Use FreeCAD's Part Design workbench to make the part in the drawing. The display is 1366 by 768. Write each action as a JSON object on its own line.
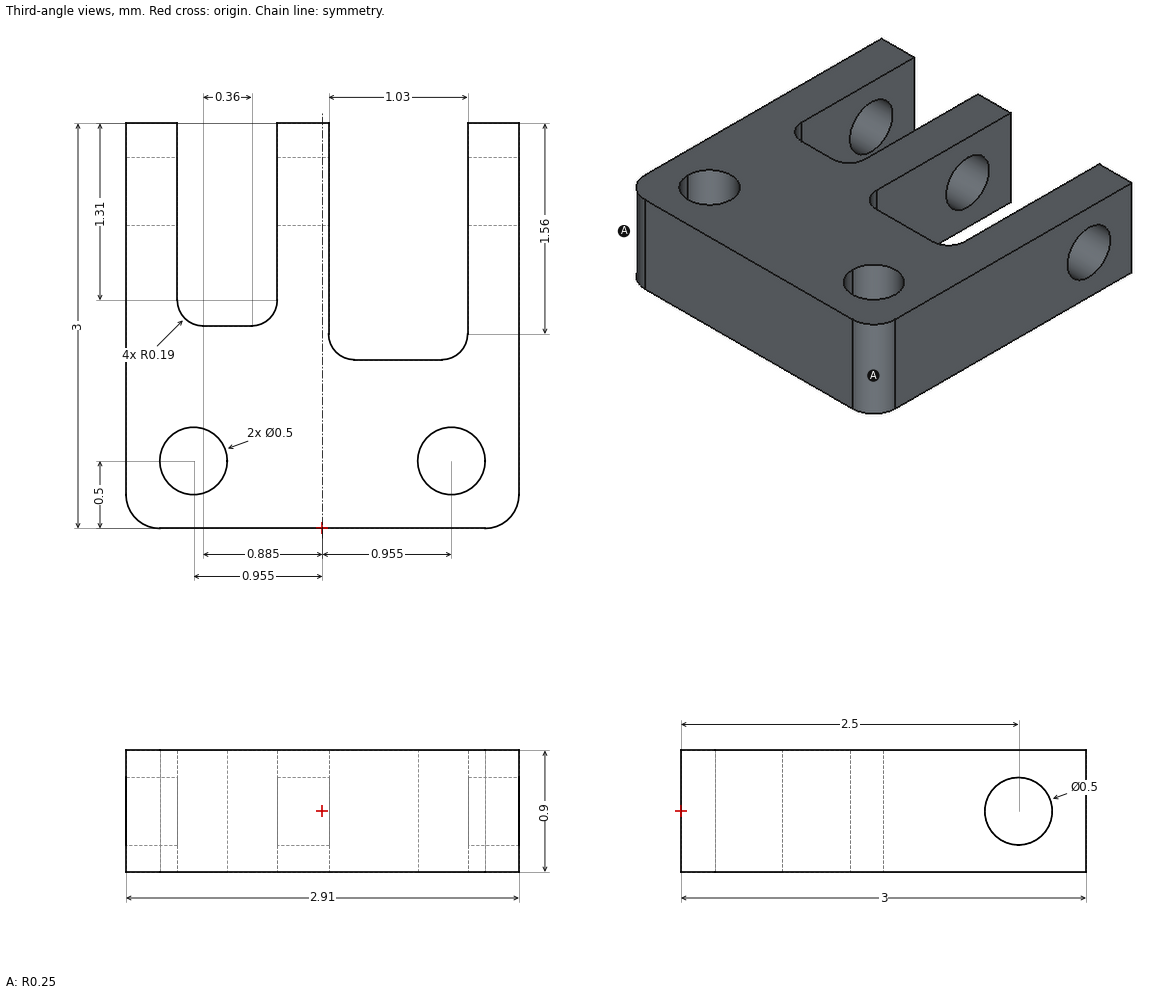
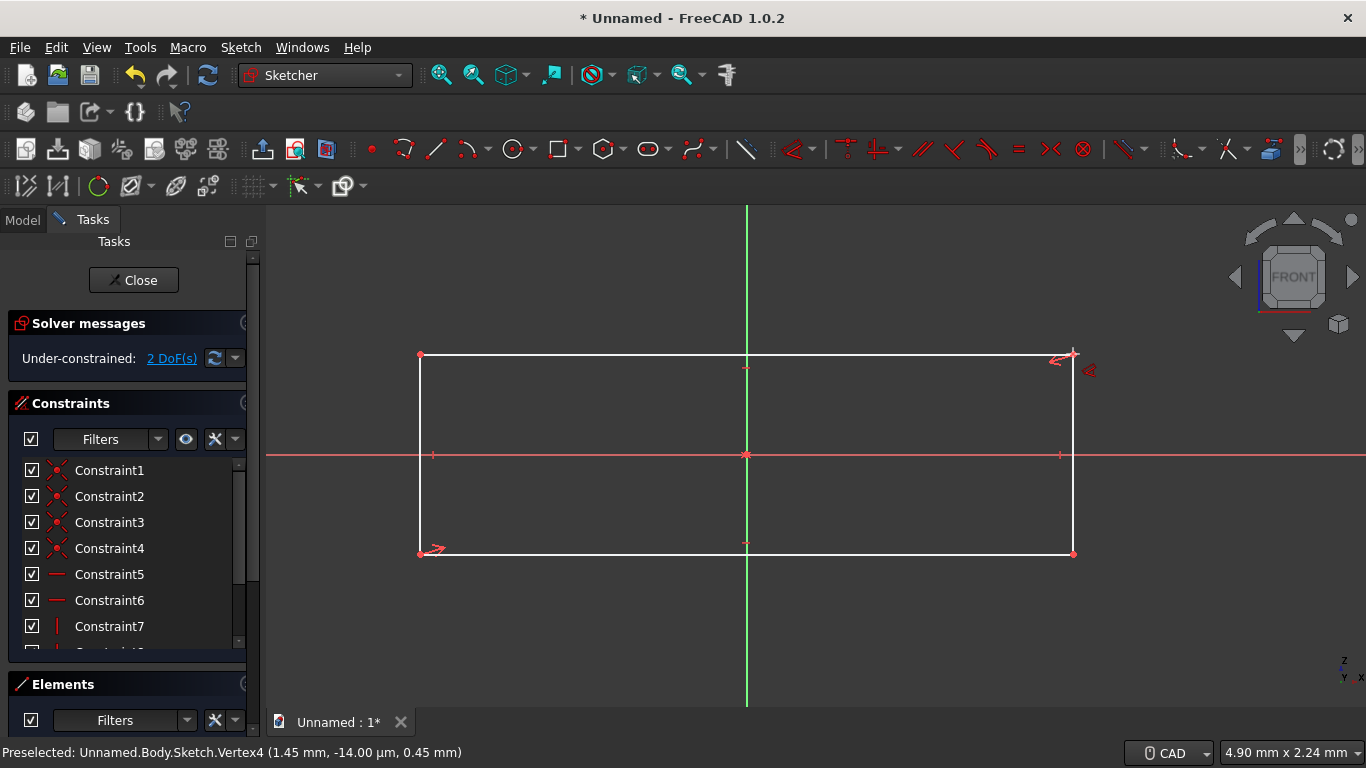
{"action": "left_click", "coordinate": [1073, 495]}
{"action": "left_click", "coordinate": [1107, 409]}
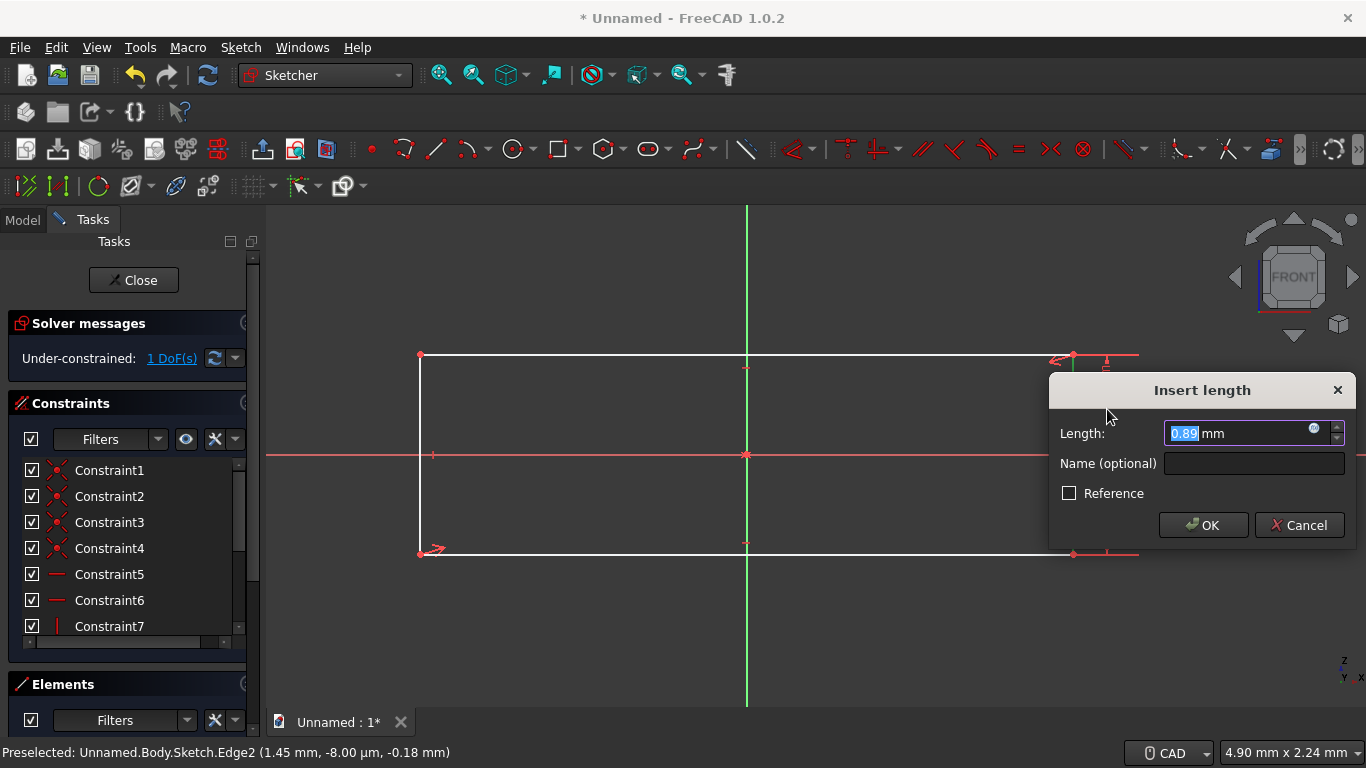
{"action": "type", "text": "0.9"}
{"action": "key", "text": "Return"}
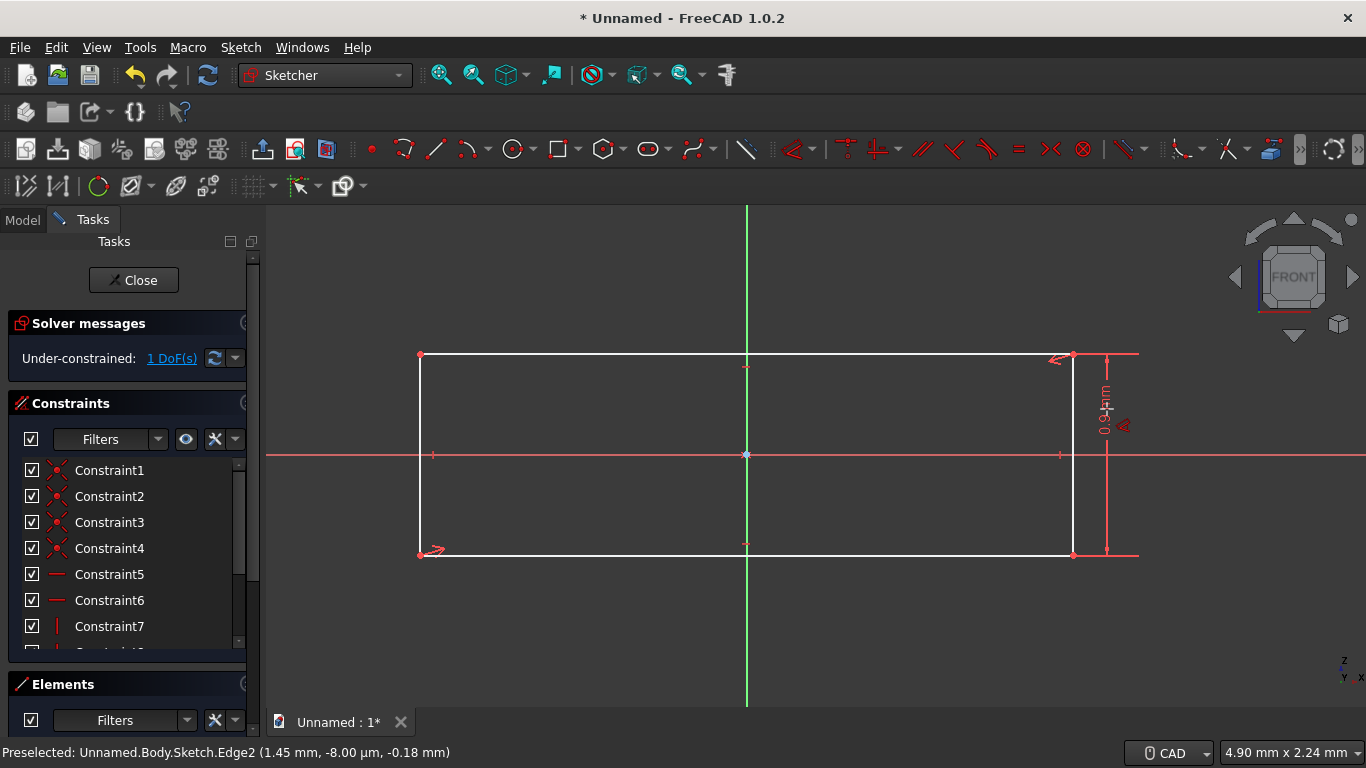
{"action": "left_click", "coordinate": [616, 556]}
{"action": "left_click", "coordinate": [597, 590]}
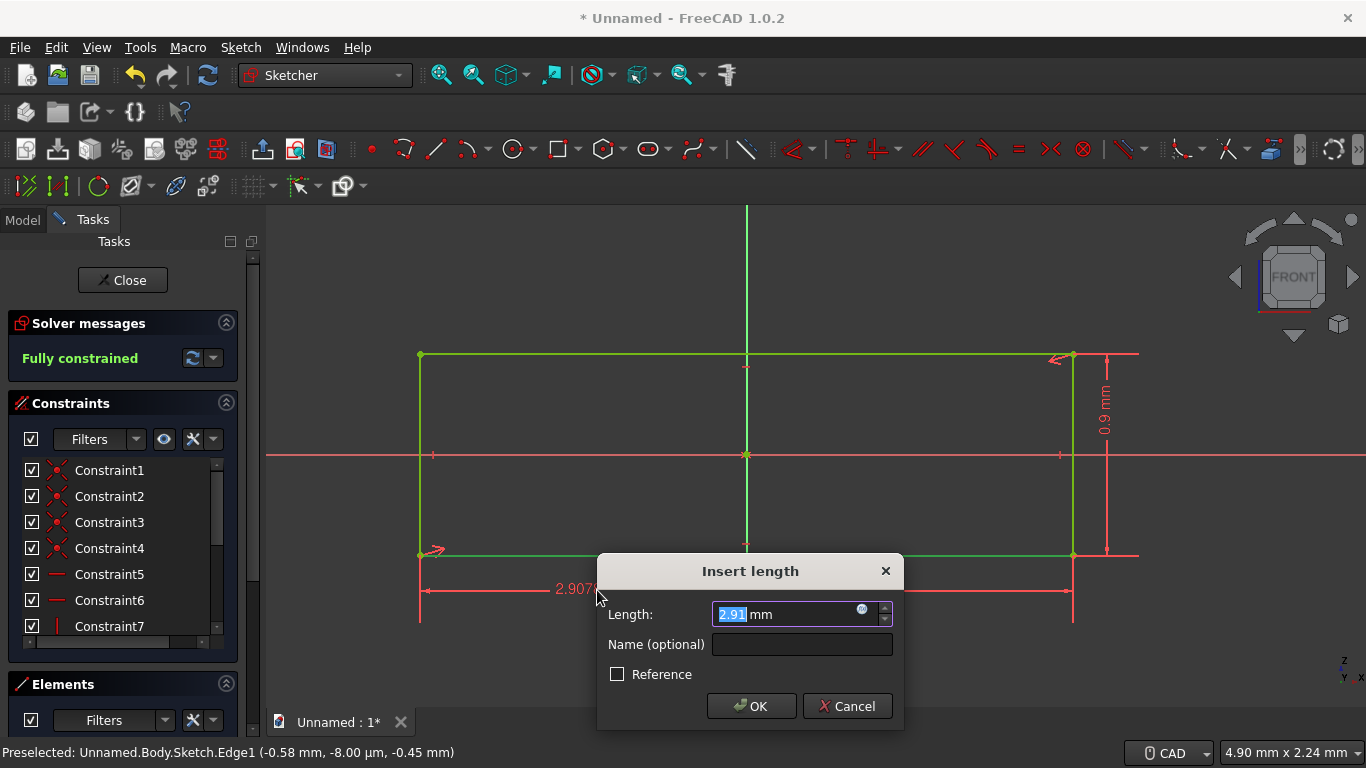
{"action": "type", "text": "2.91"}
{"action": "key", "text": "Return"}
{"action": "key", "text": "Escape"}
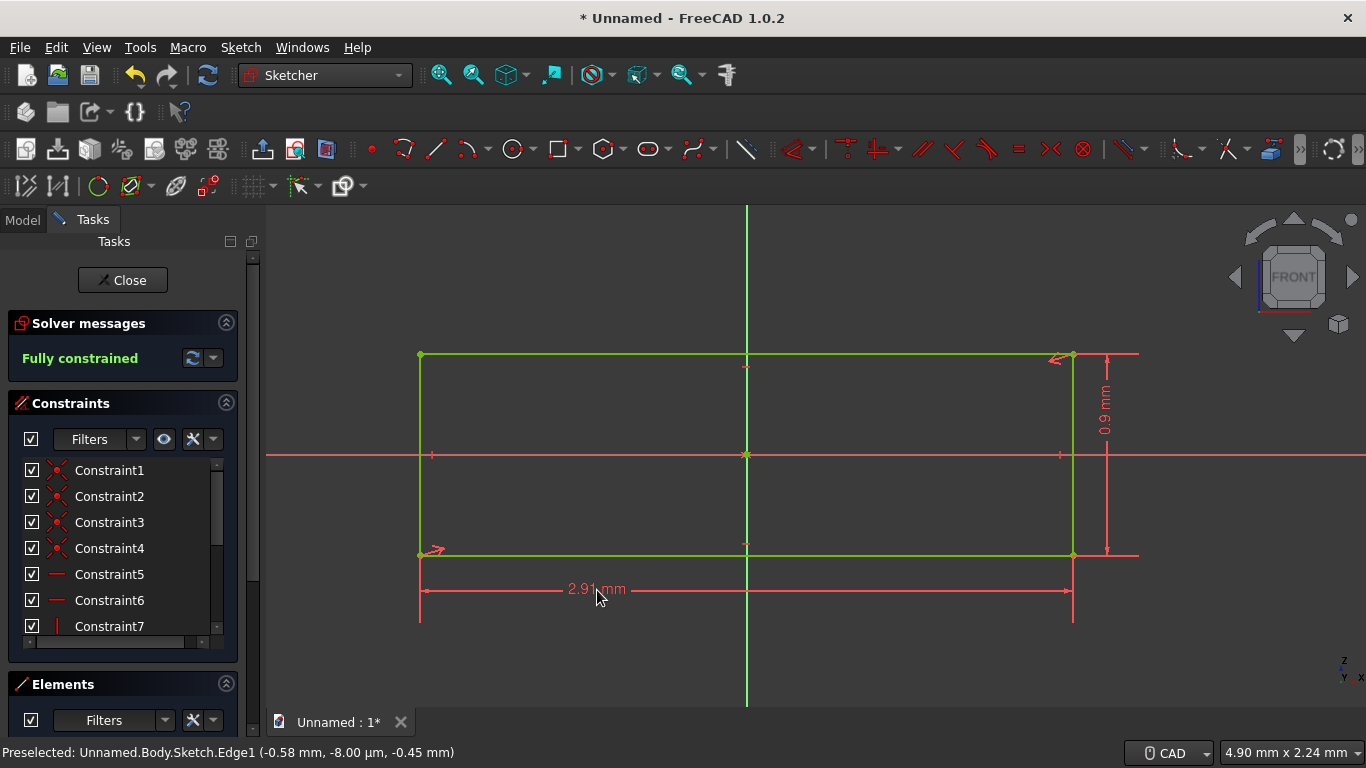
{"action": "left_click", "coordinate": [123, 280]}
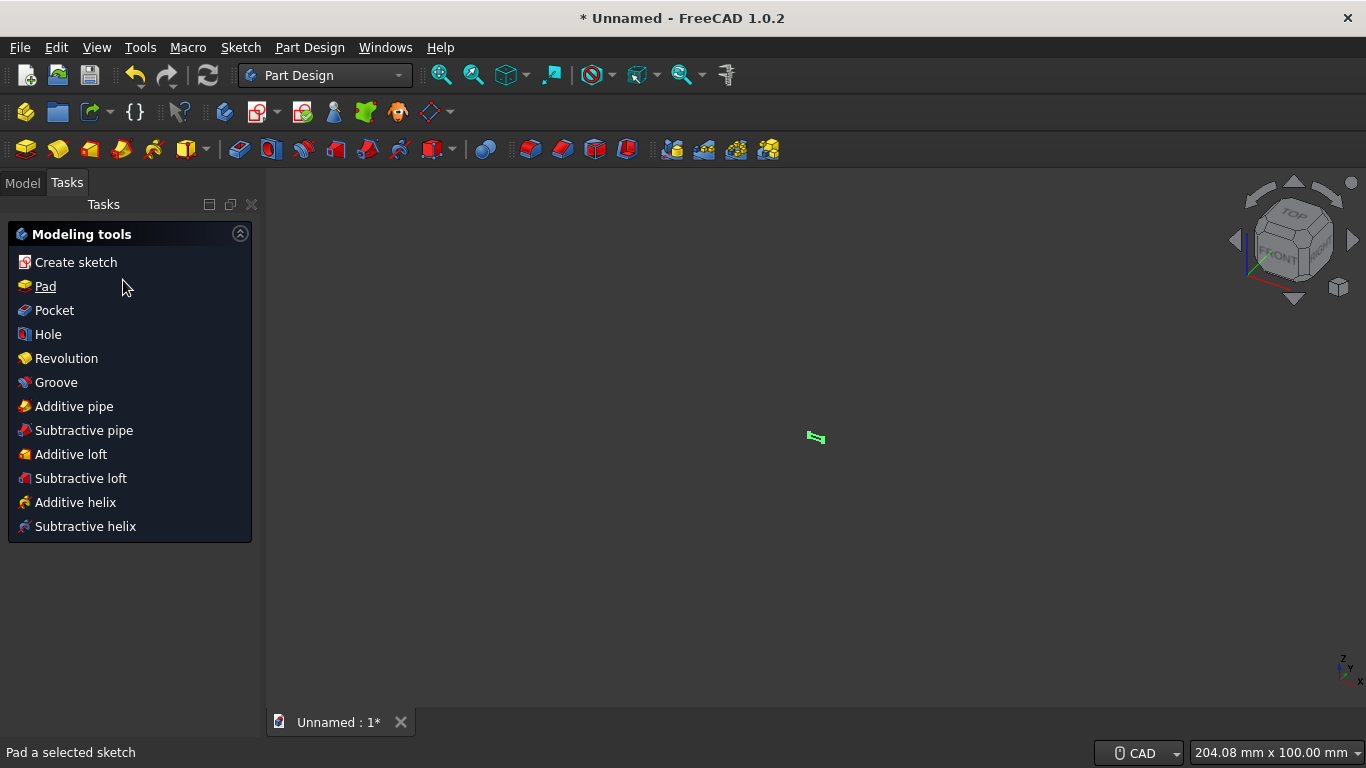
{"action": "left_click", "coordinate": [26, 150]}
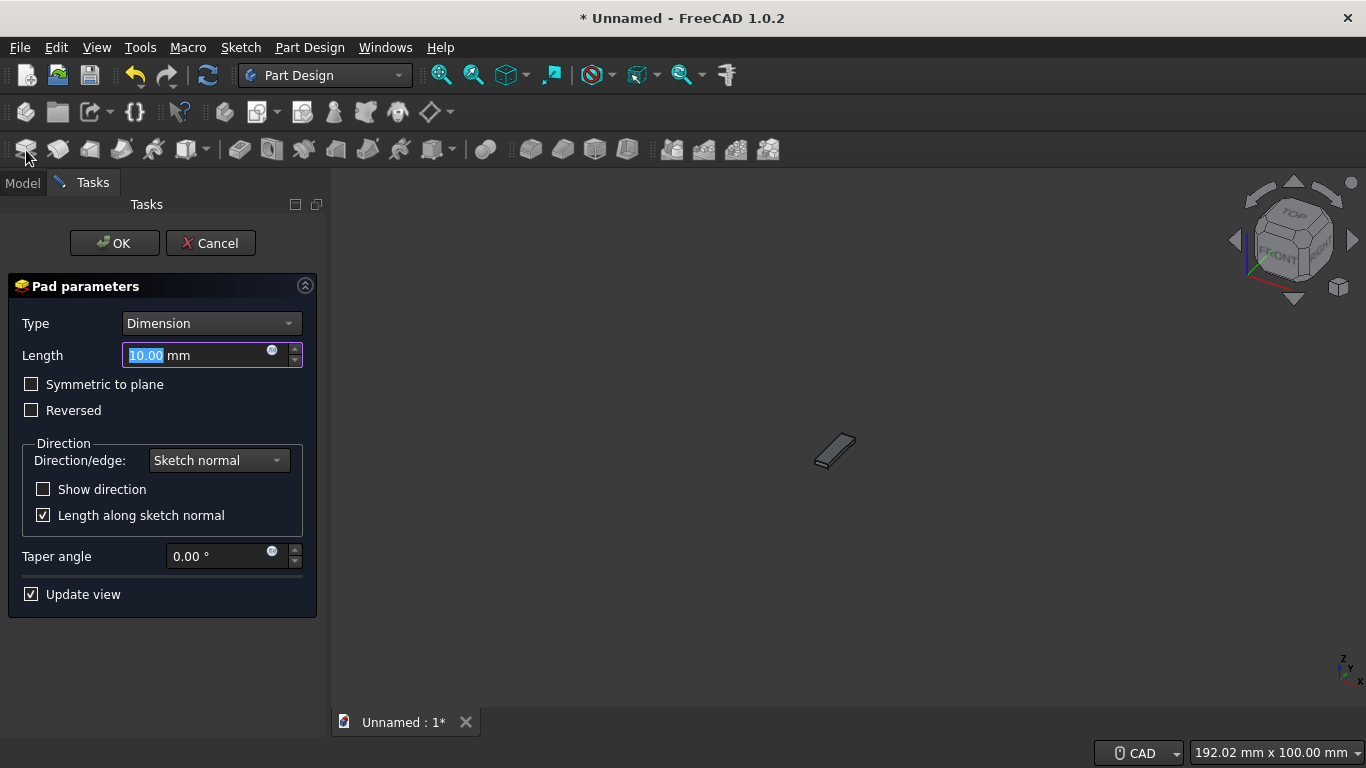
{"action": "type", "text": "3"}
{"action": "key", "text": "Tab"}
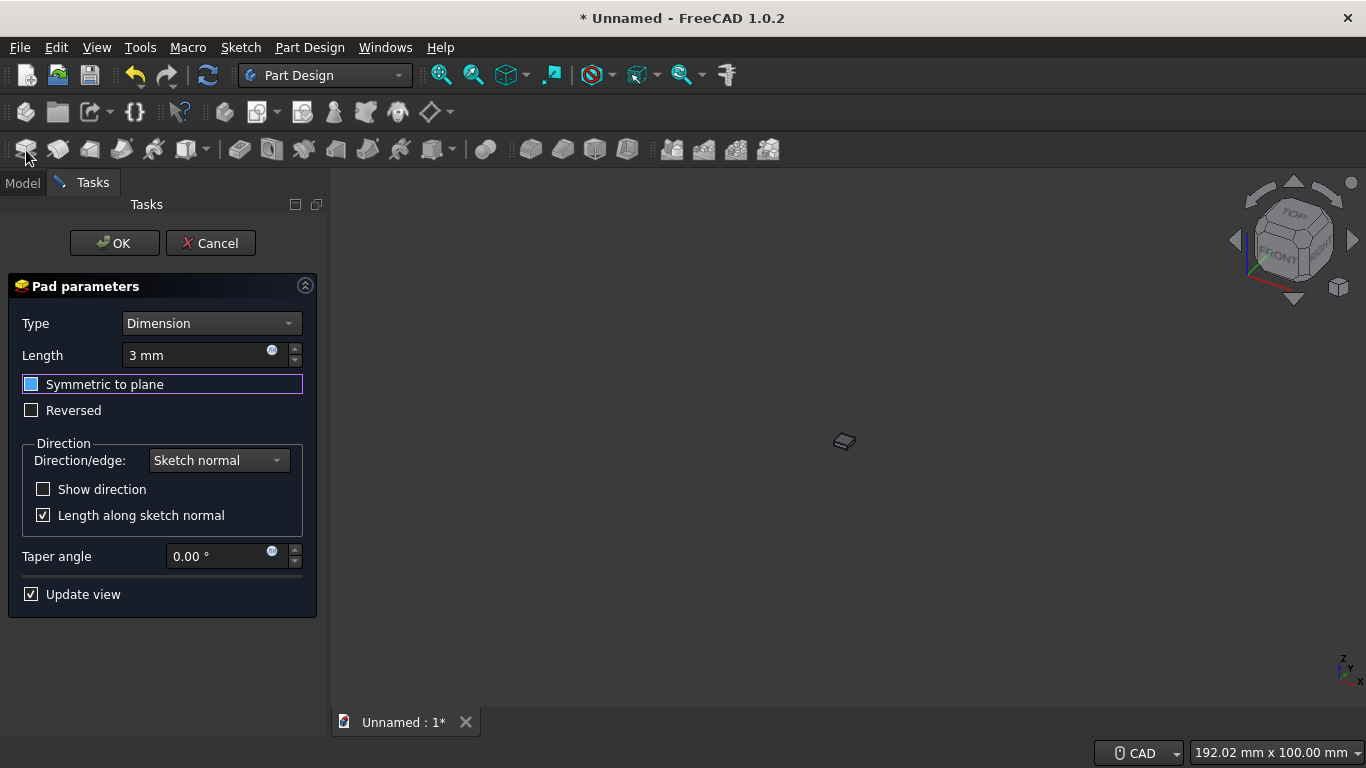
{"action": "left_click", "coordinate": [30, 410]}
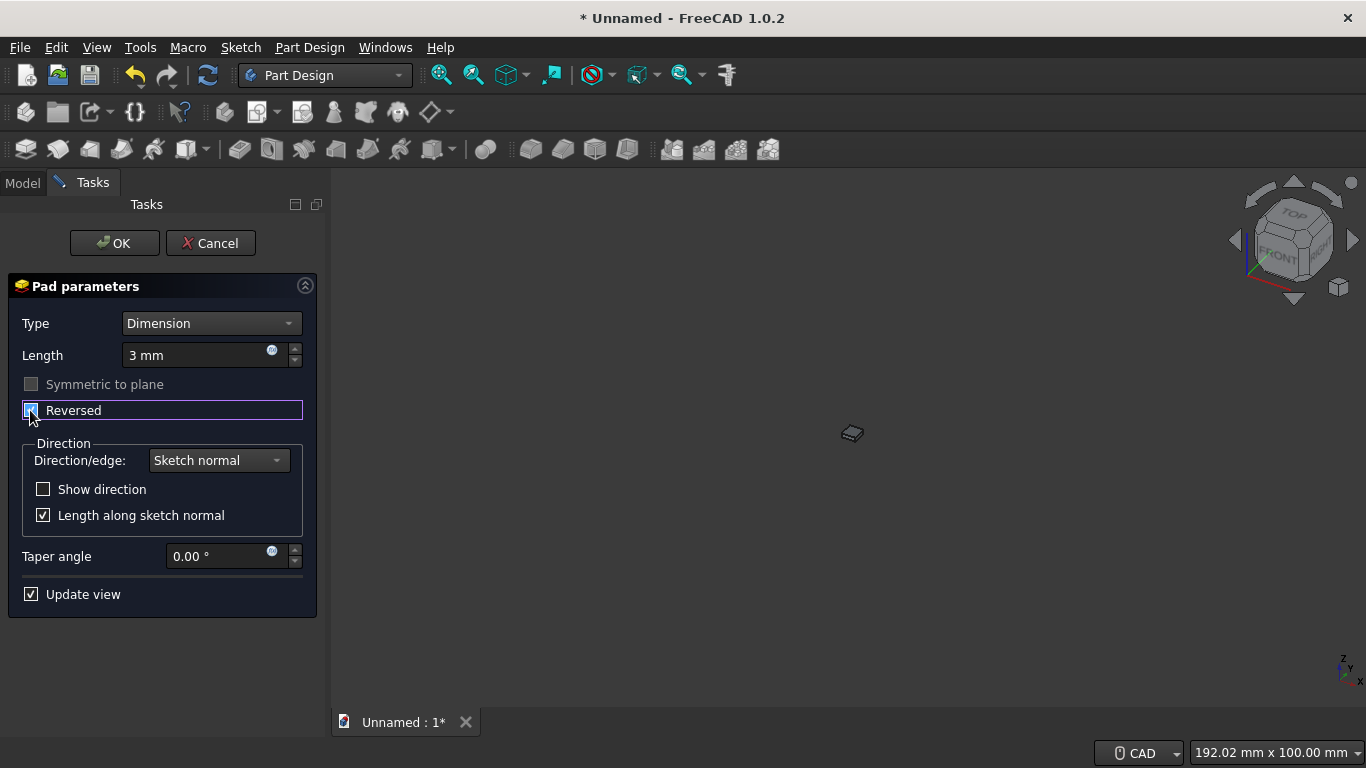
{"action": "left_click", "coordinate": [115, 243]}